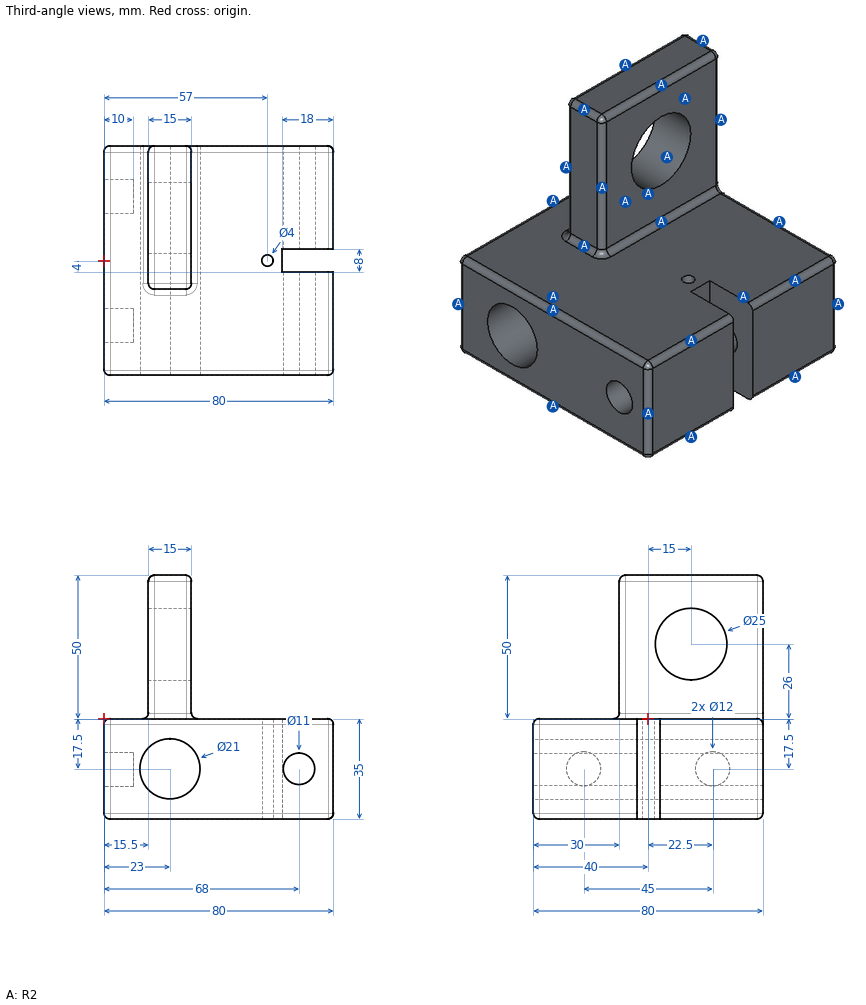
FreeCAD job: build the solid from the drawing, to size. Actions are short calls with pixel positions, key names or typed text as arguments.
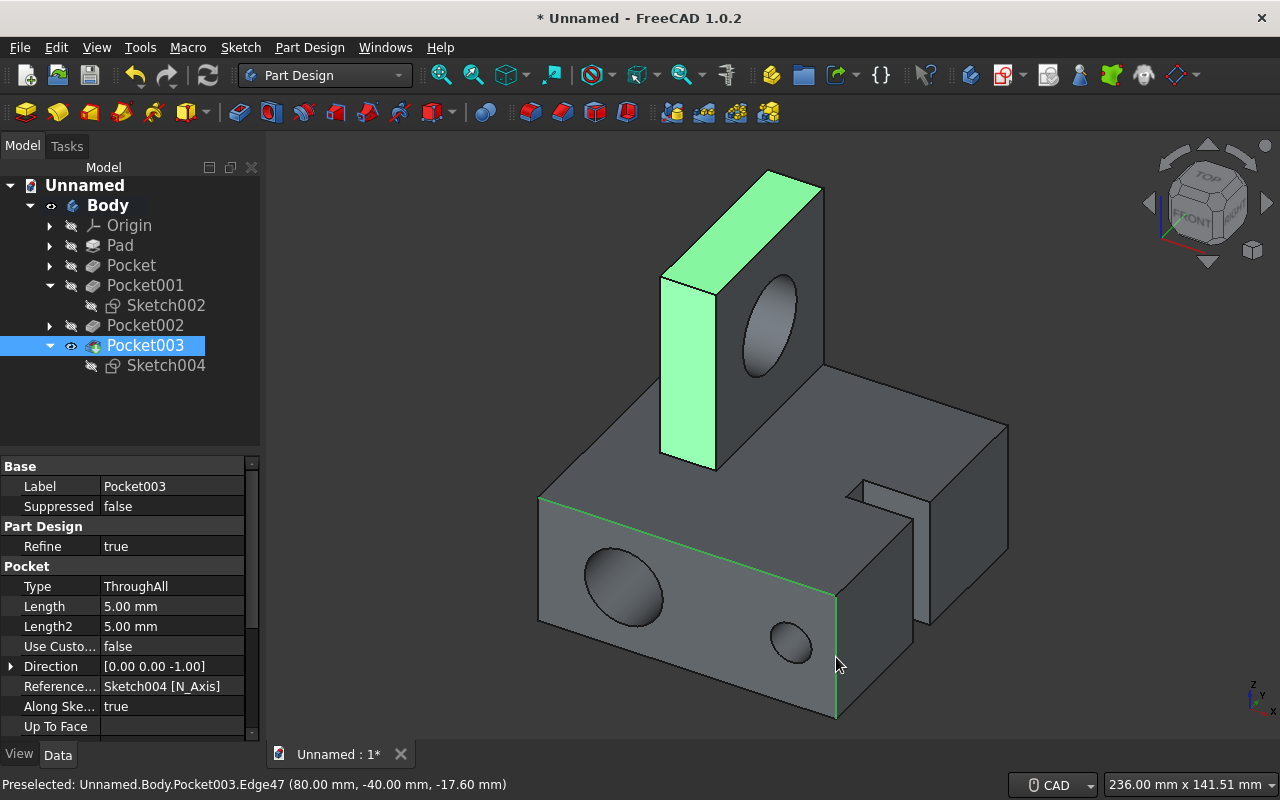
click(969, 463, ctrl)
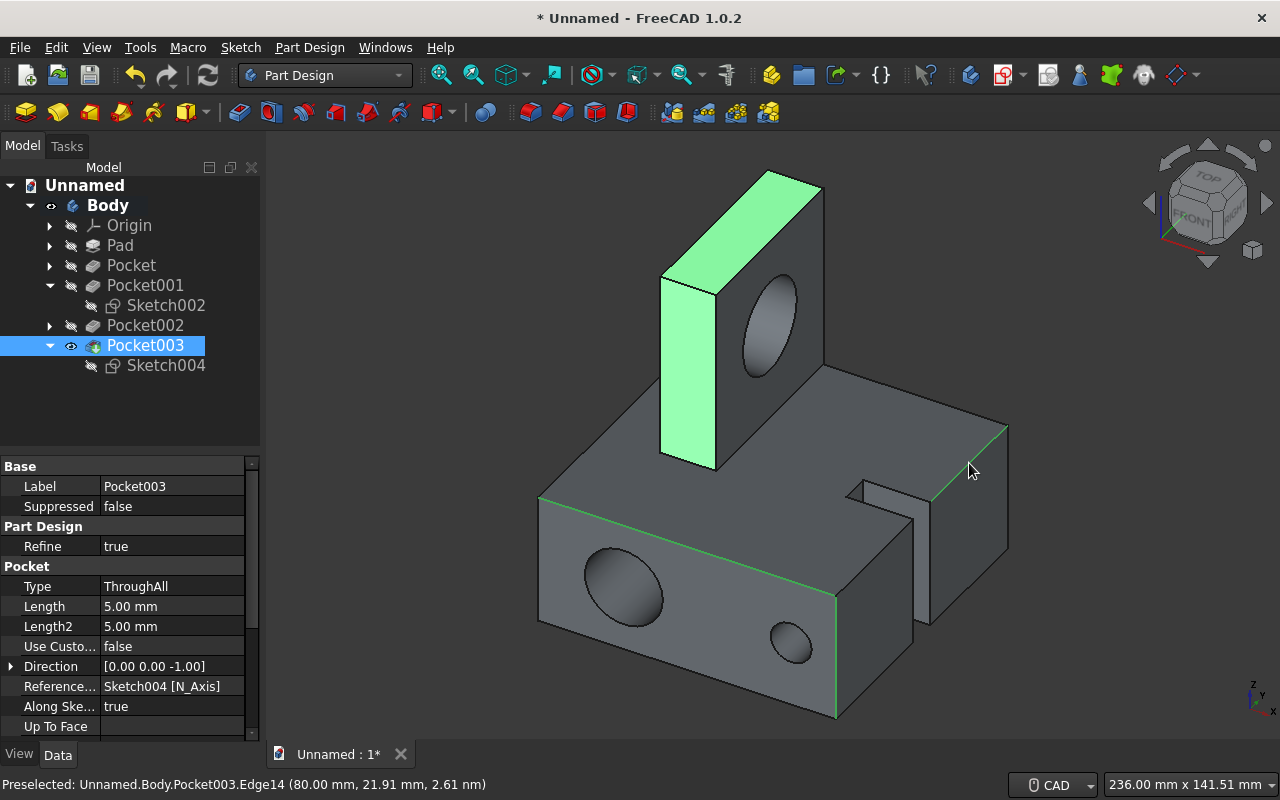
click(875, 557, ctrl)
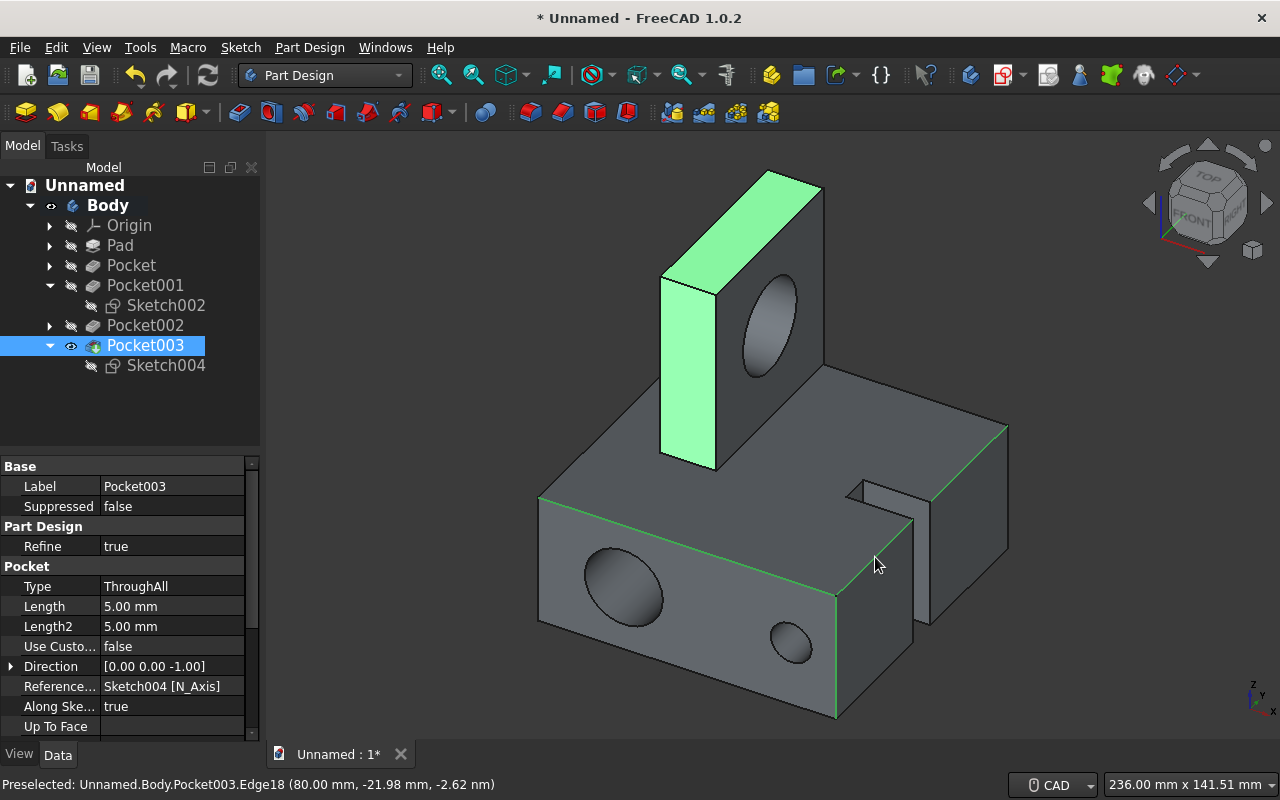
key(0)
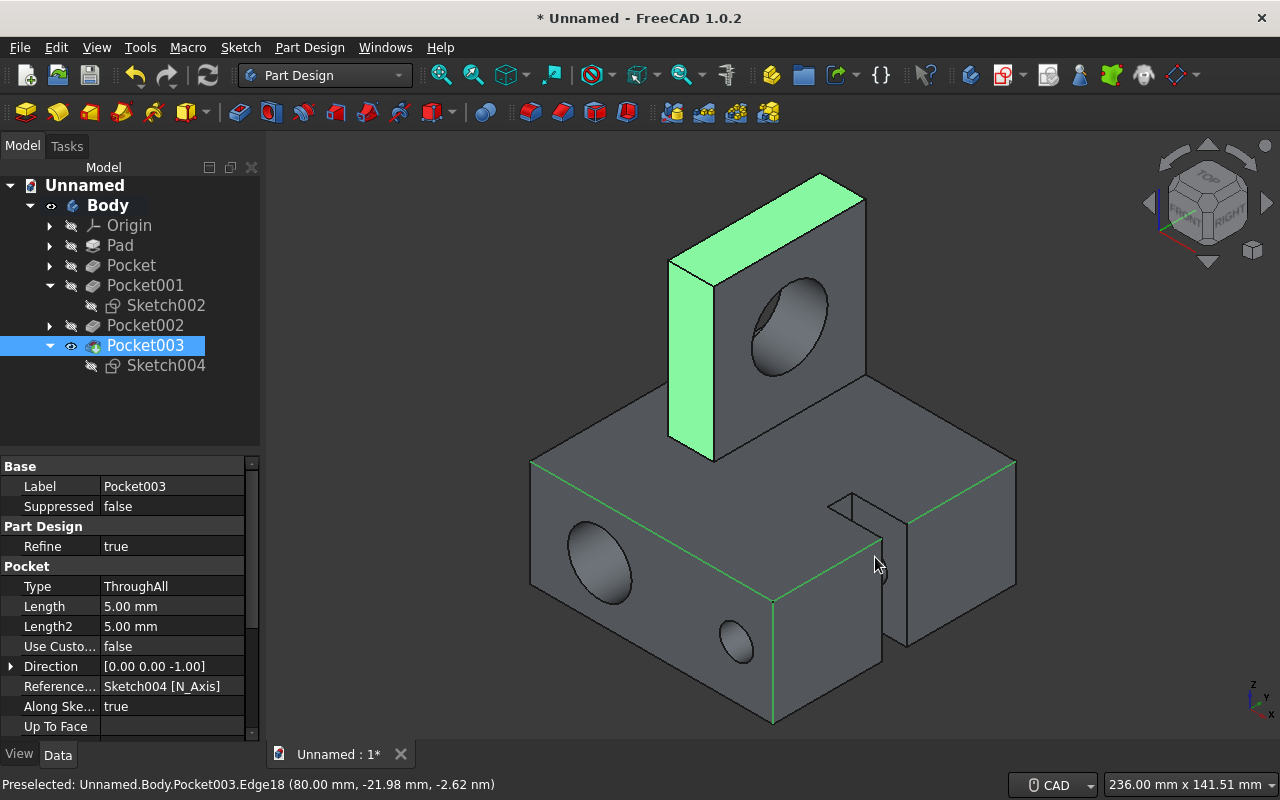
key(2)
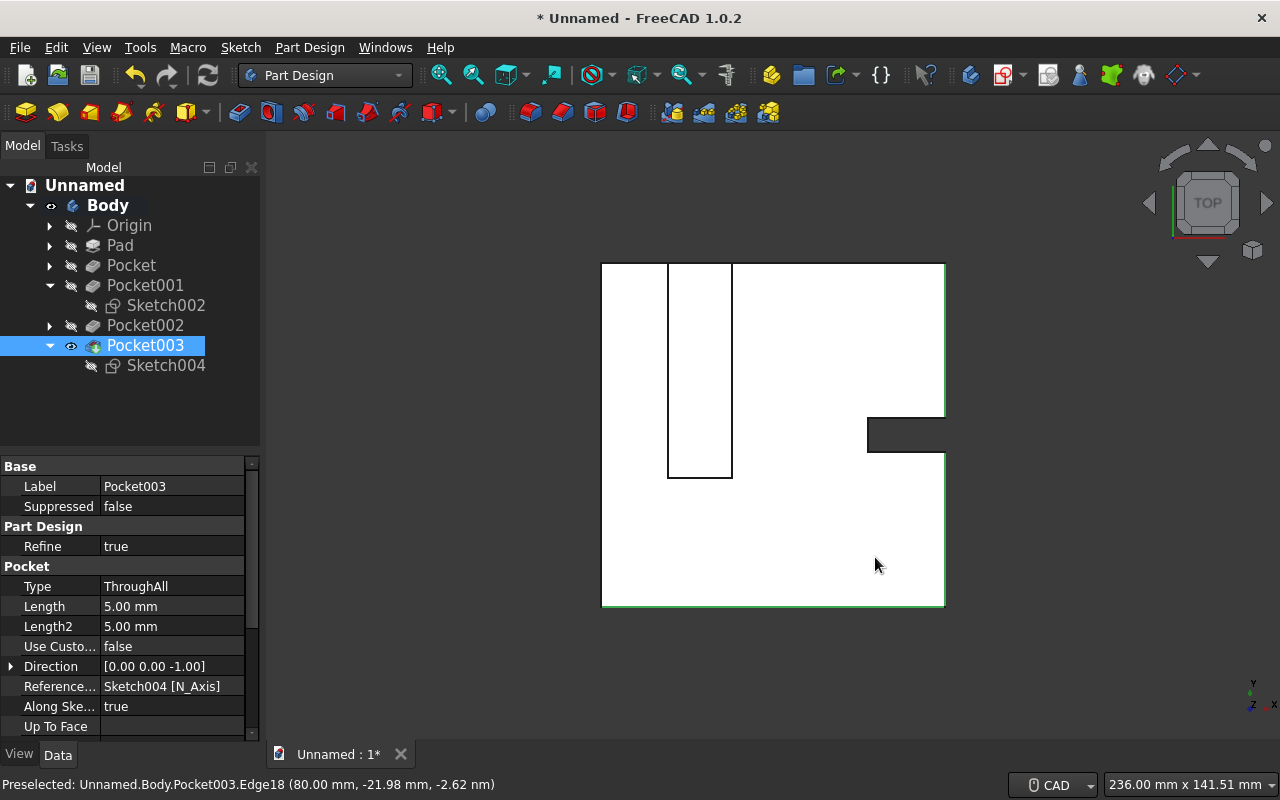
click(839, 262, ctrl)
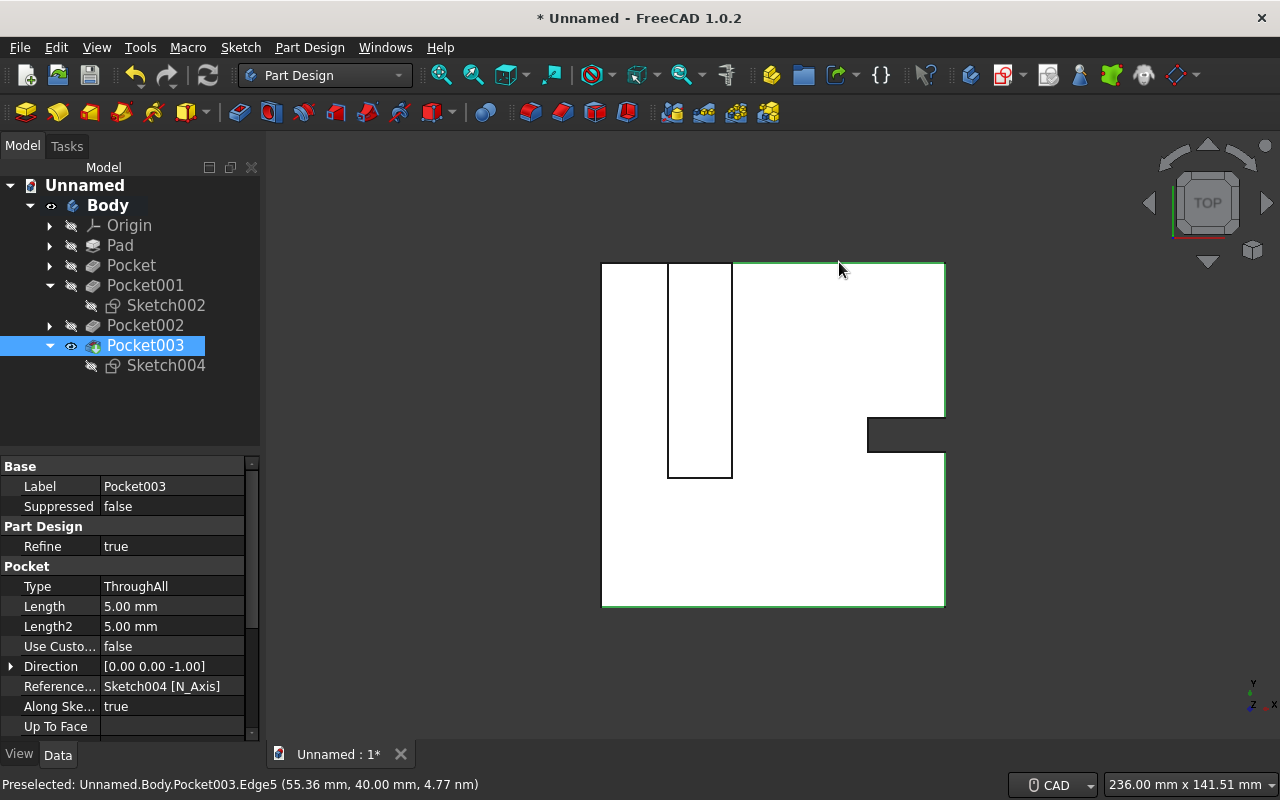
click(601, 434, ctrl)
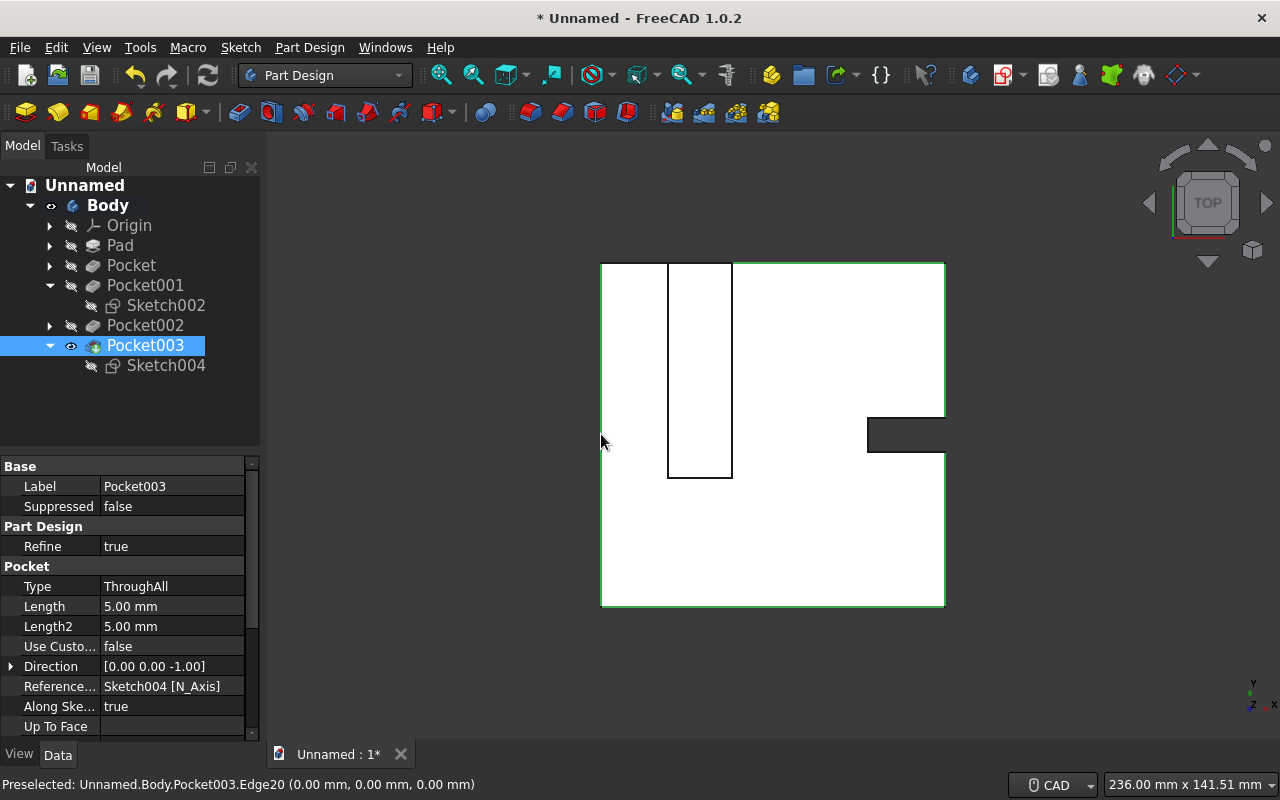
click(634, 262, ctrl)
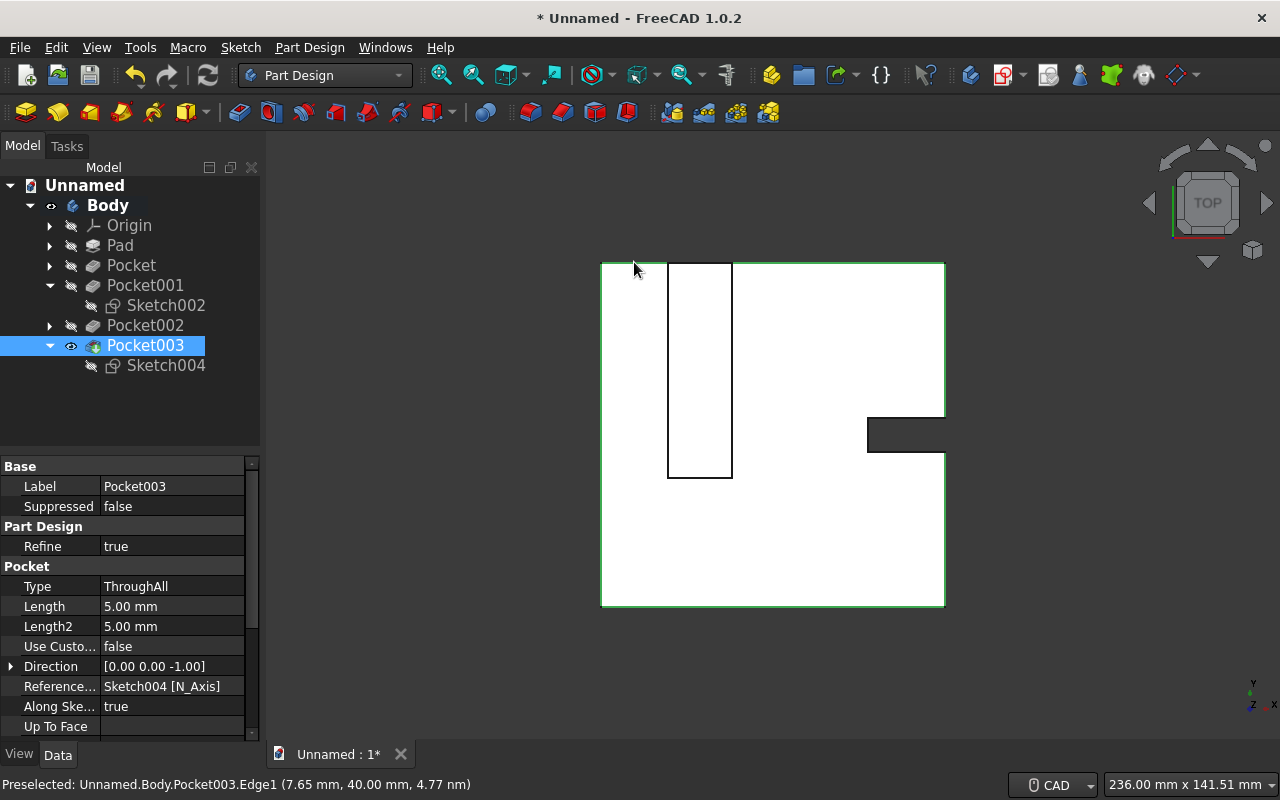
key(1)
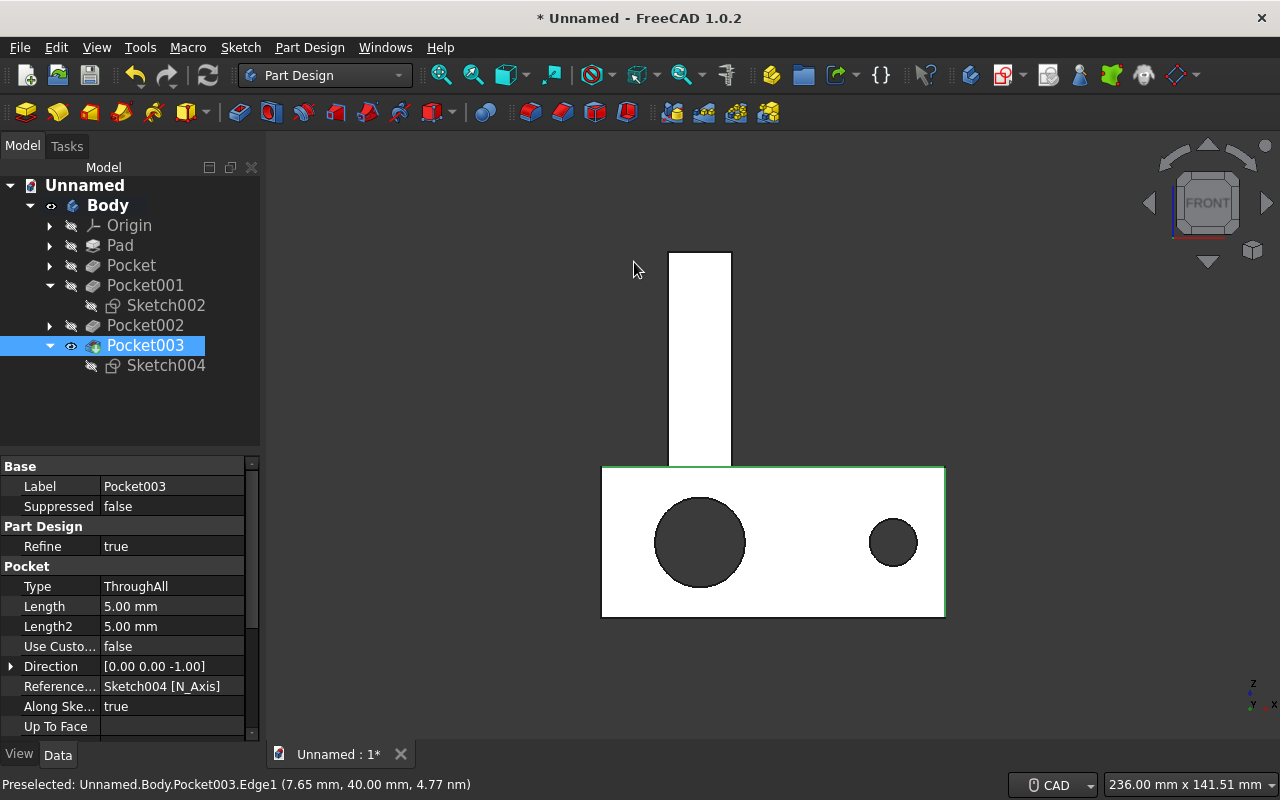
click(601, 541, ctrl)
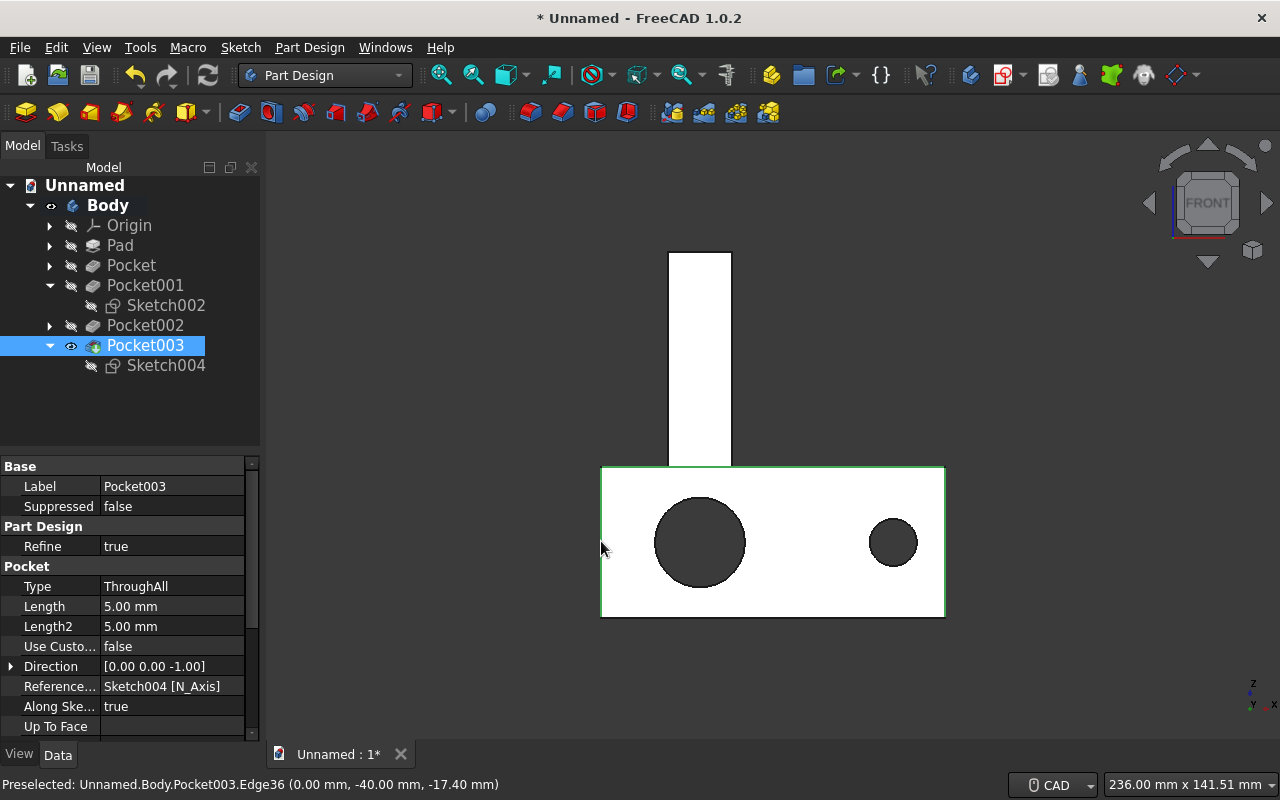
key(3)